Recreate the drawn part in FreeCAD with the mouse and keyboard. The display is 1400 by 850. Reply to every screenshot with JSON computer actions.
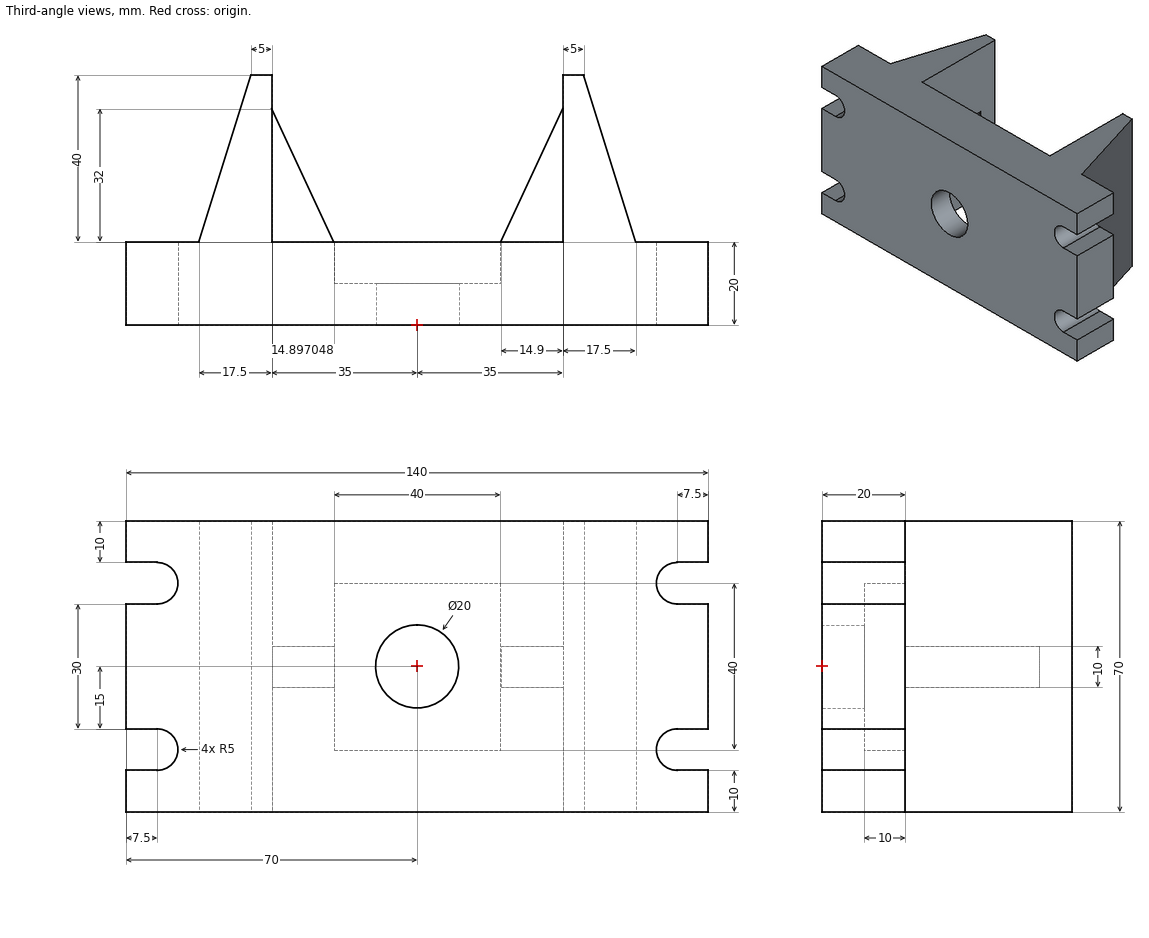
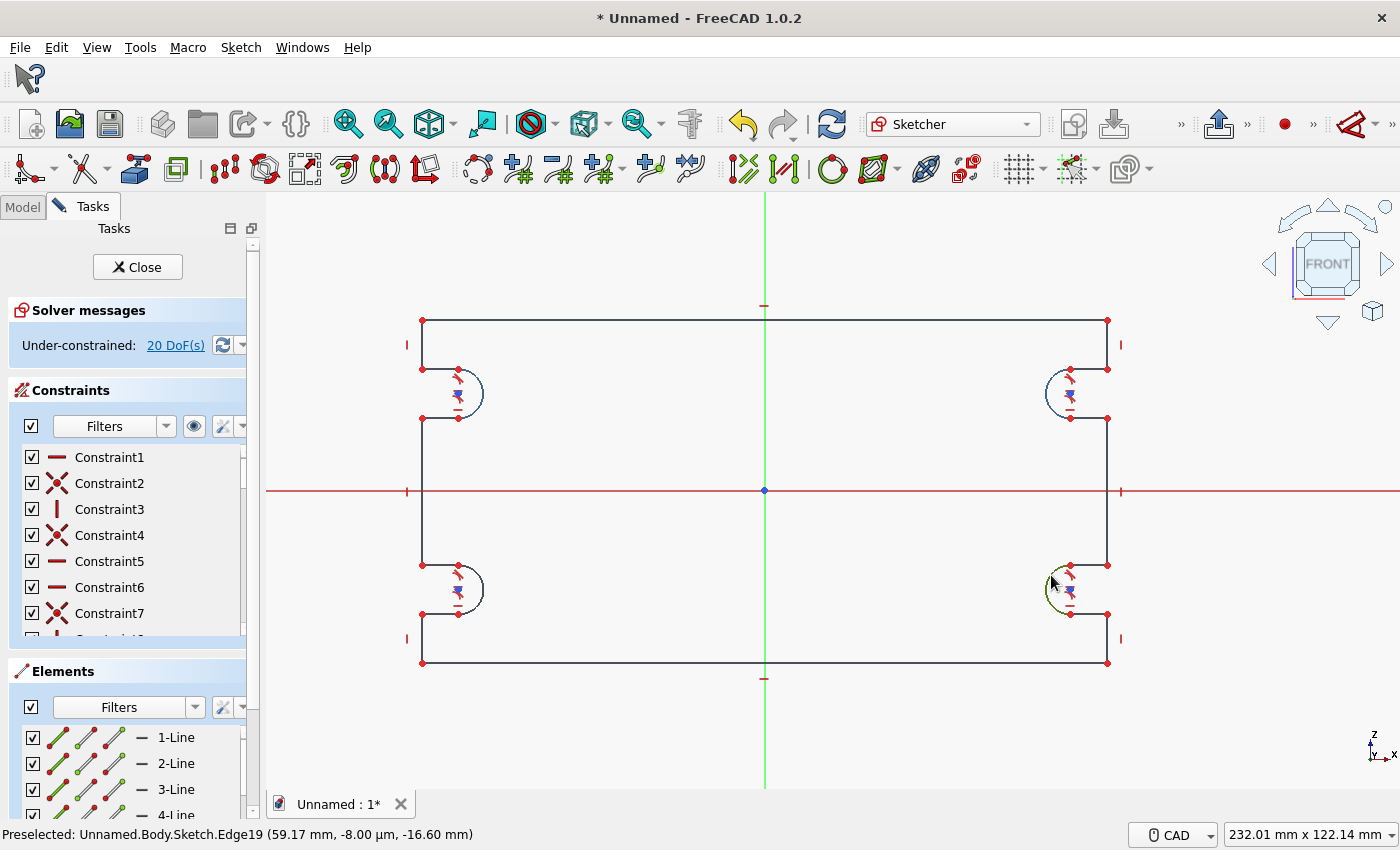
{"action": "left_click", "coordinate": [479, 604]}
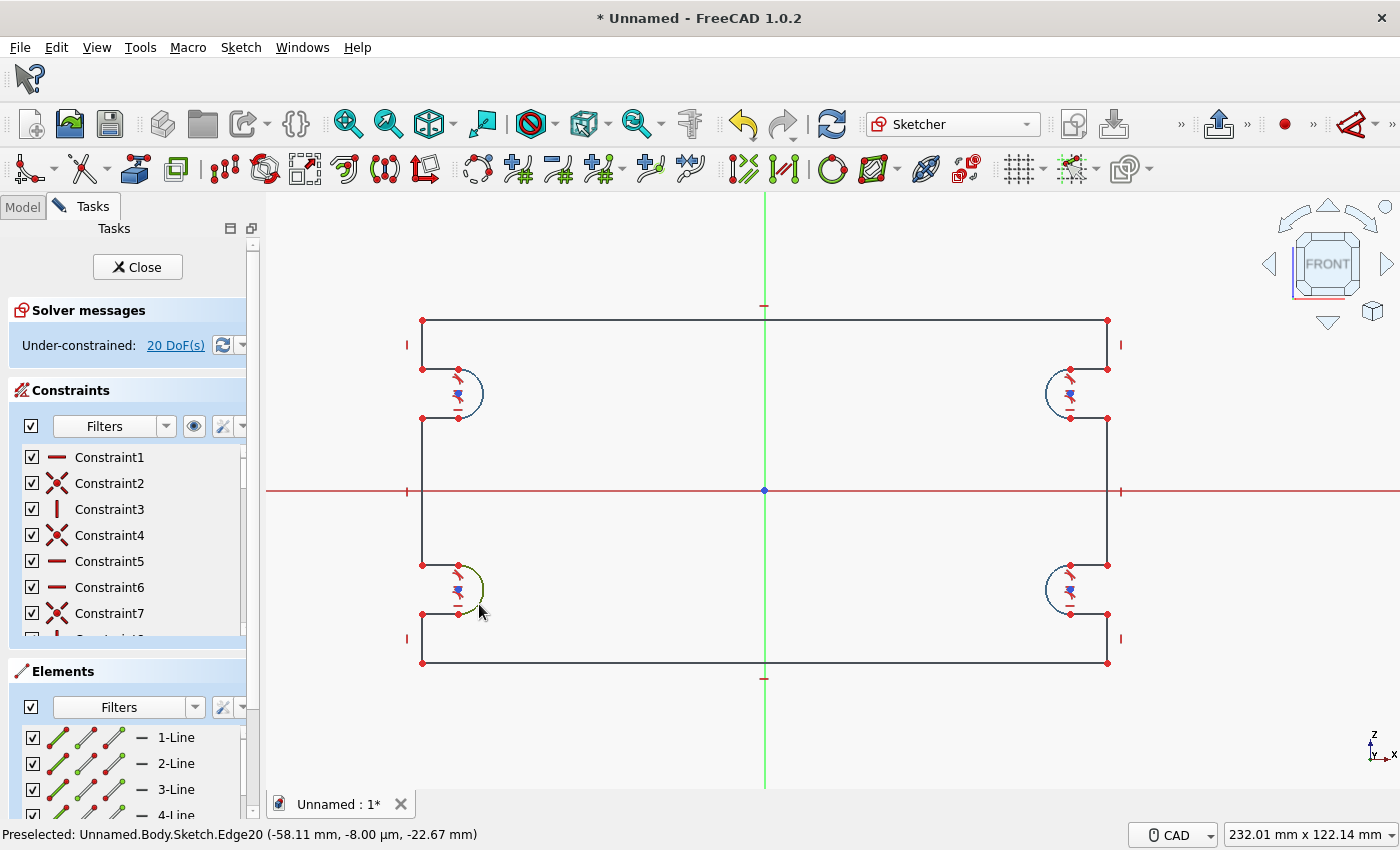
{"action": "key", "text": "e"}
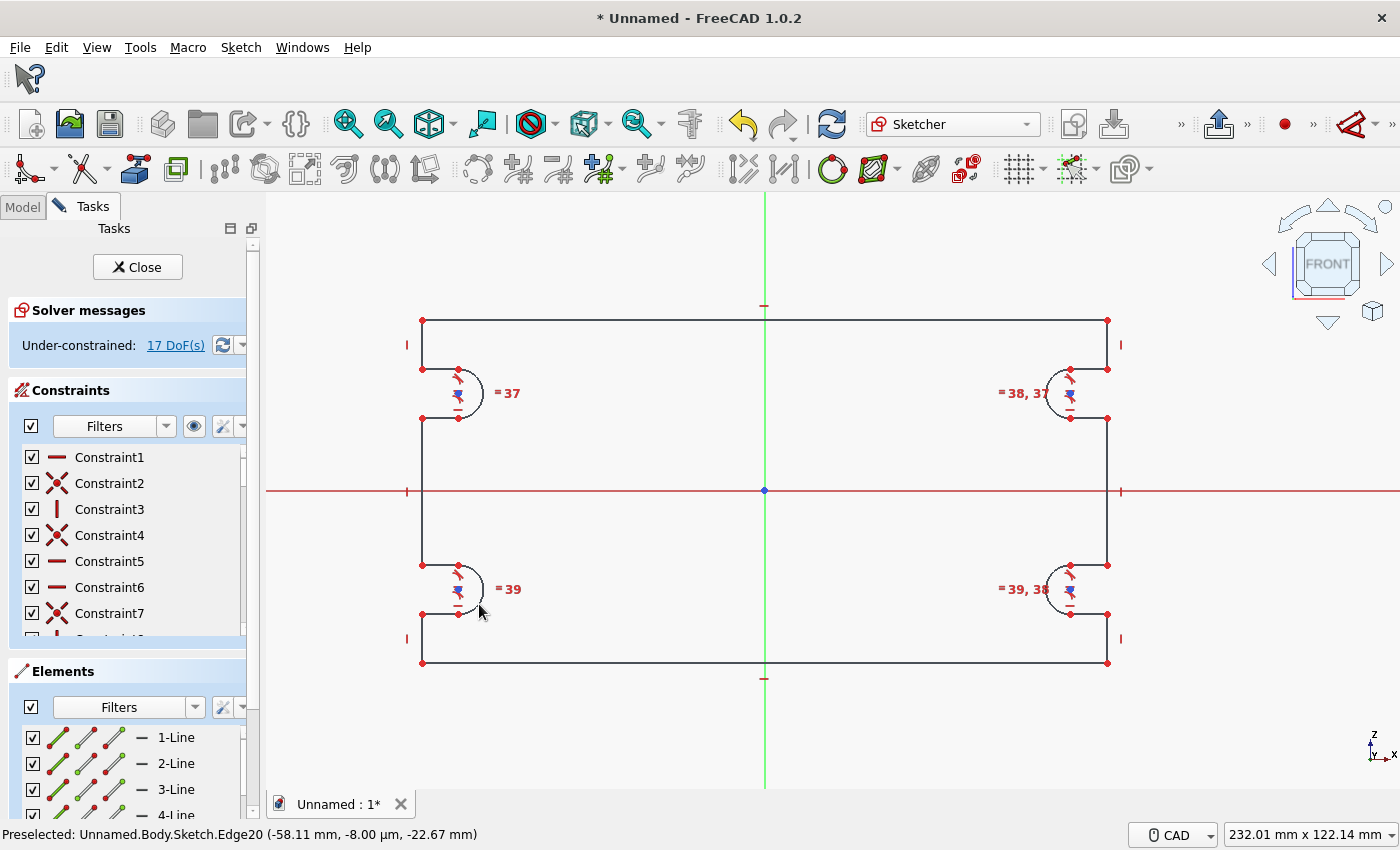
{"action": "scroll", "coordinate": [478, 408], "scroll_direction": "up", "scroll_amount": 3}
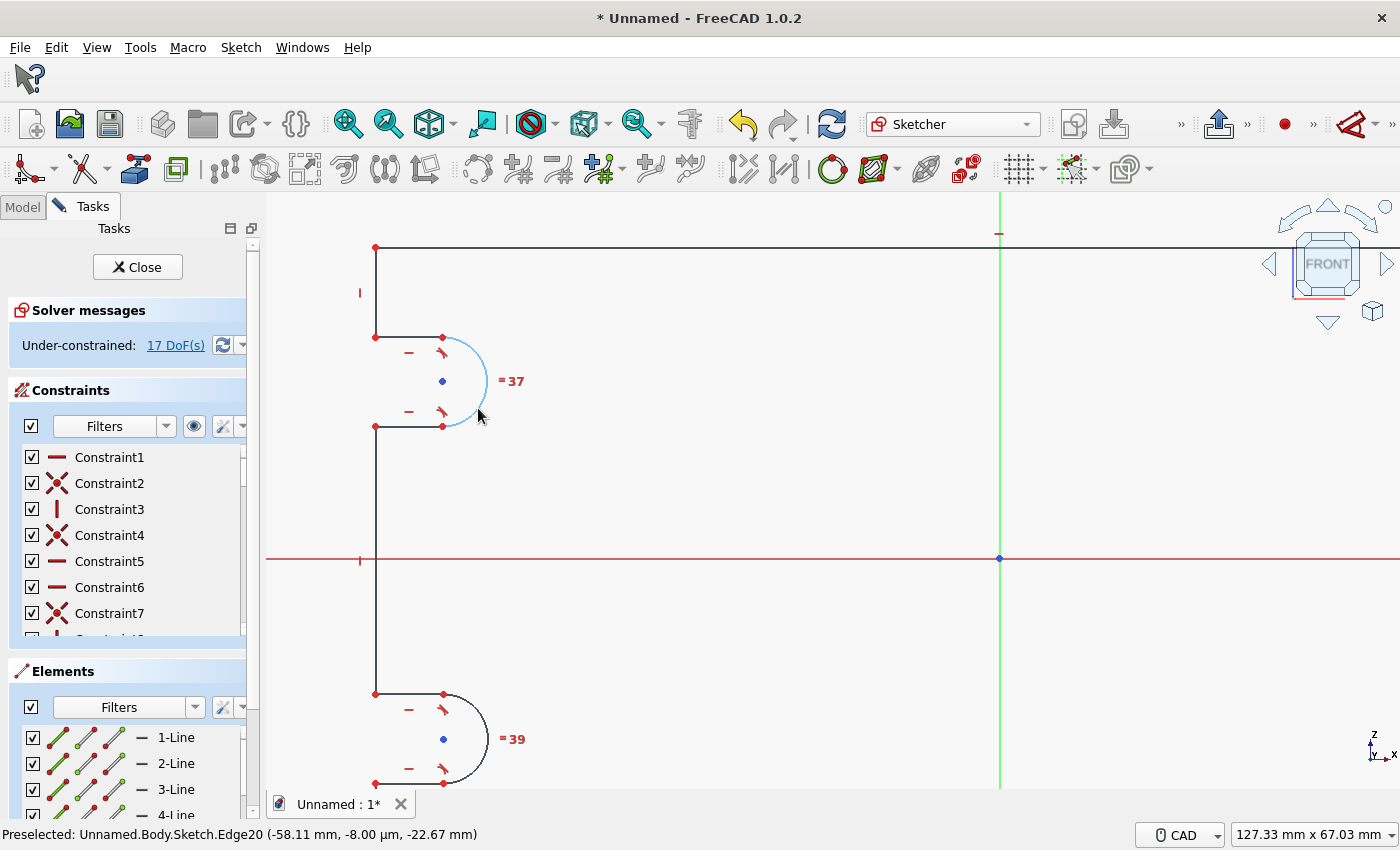
{"action": "left_click", "coordinate": [478, 408]}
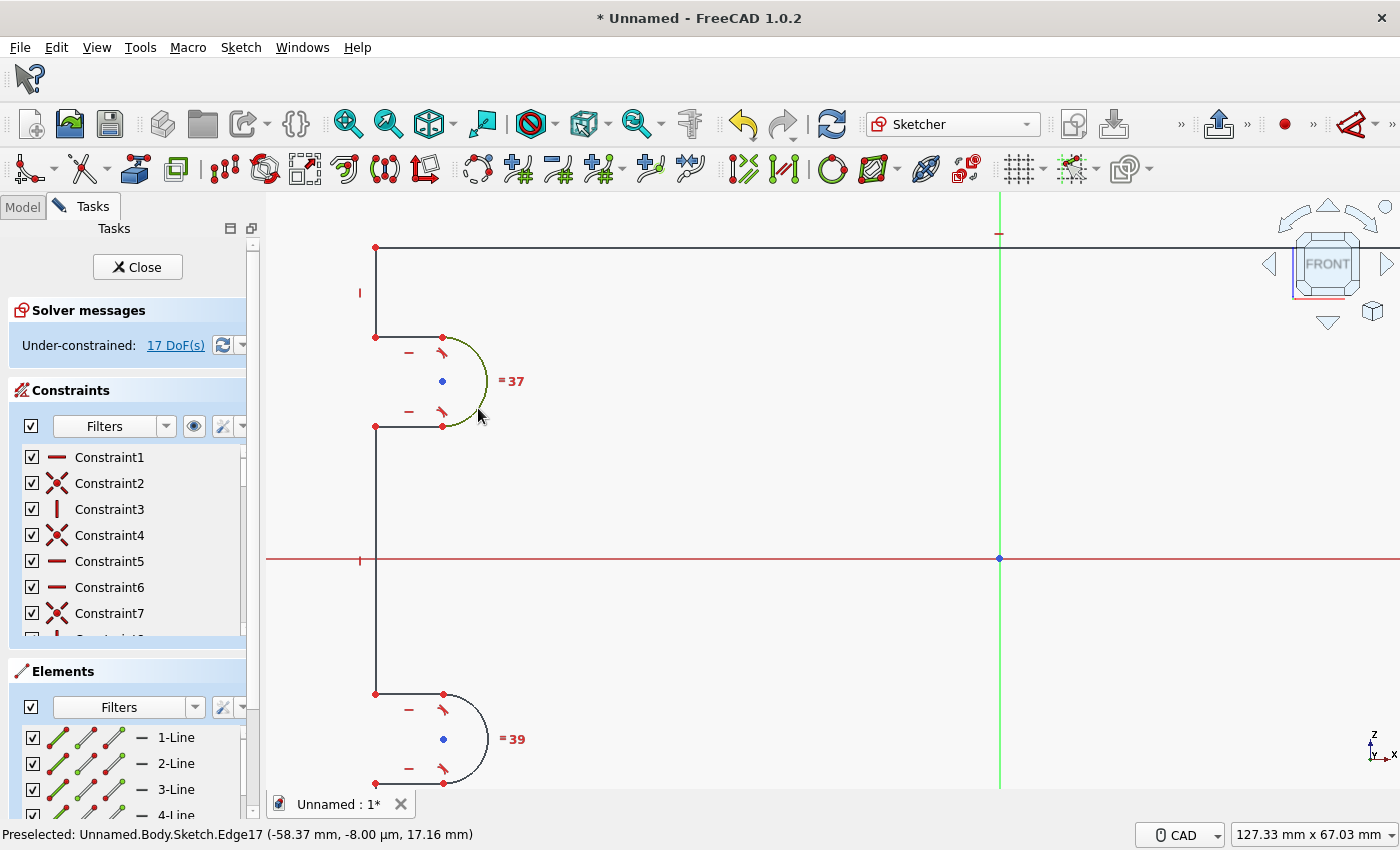
{"action": "left_click", "coordinate": [1378, 124]}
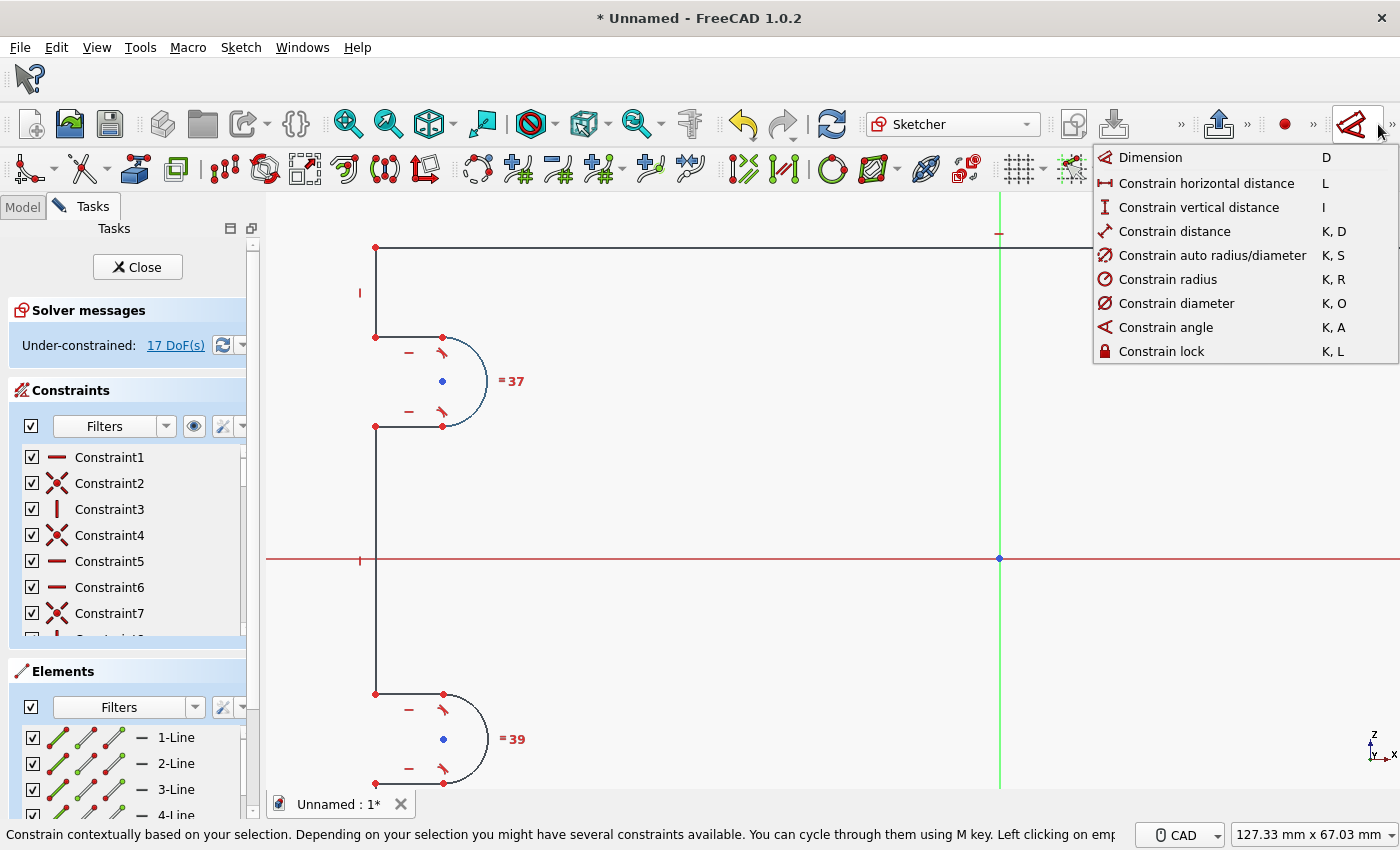
{"action": "left_click", "coordinate": [1246, 279]}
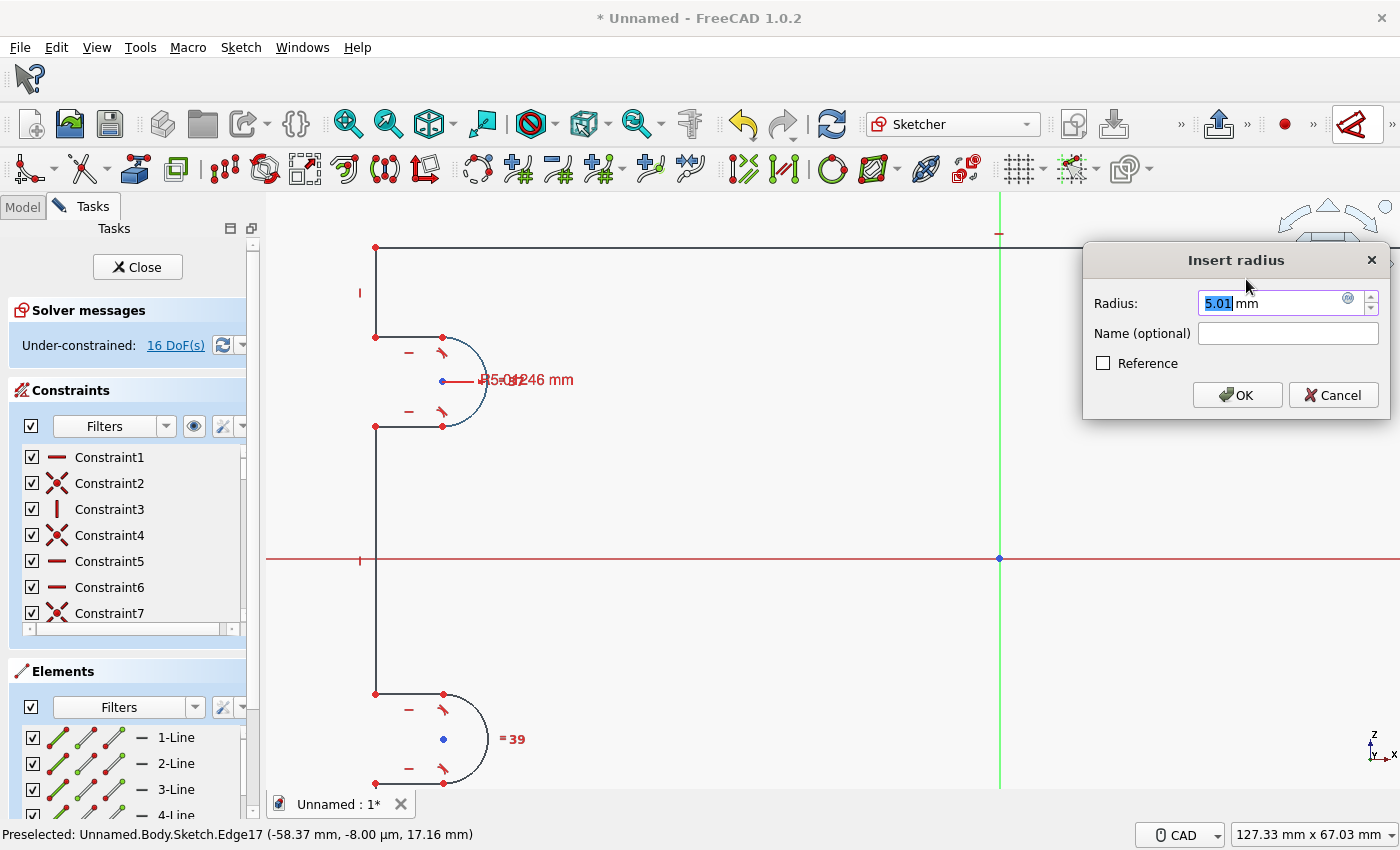
{"action": "type", "text": "5"}
{"action": "key", "text": "Return"}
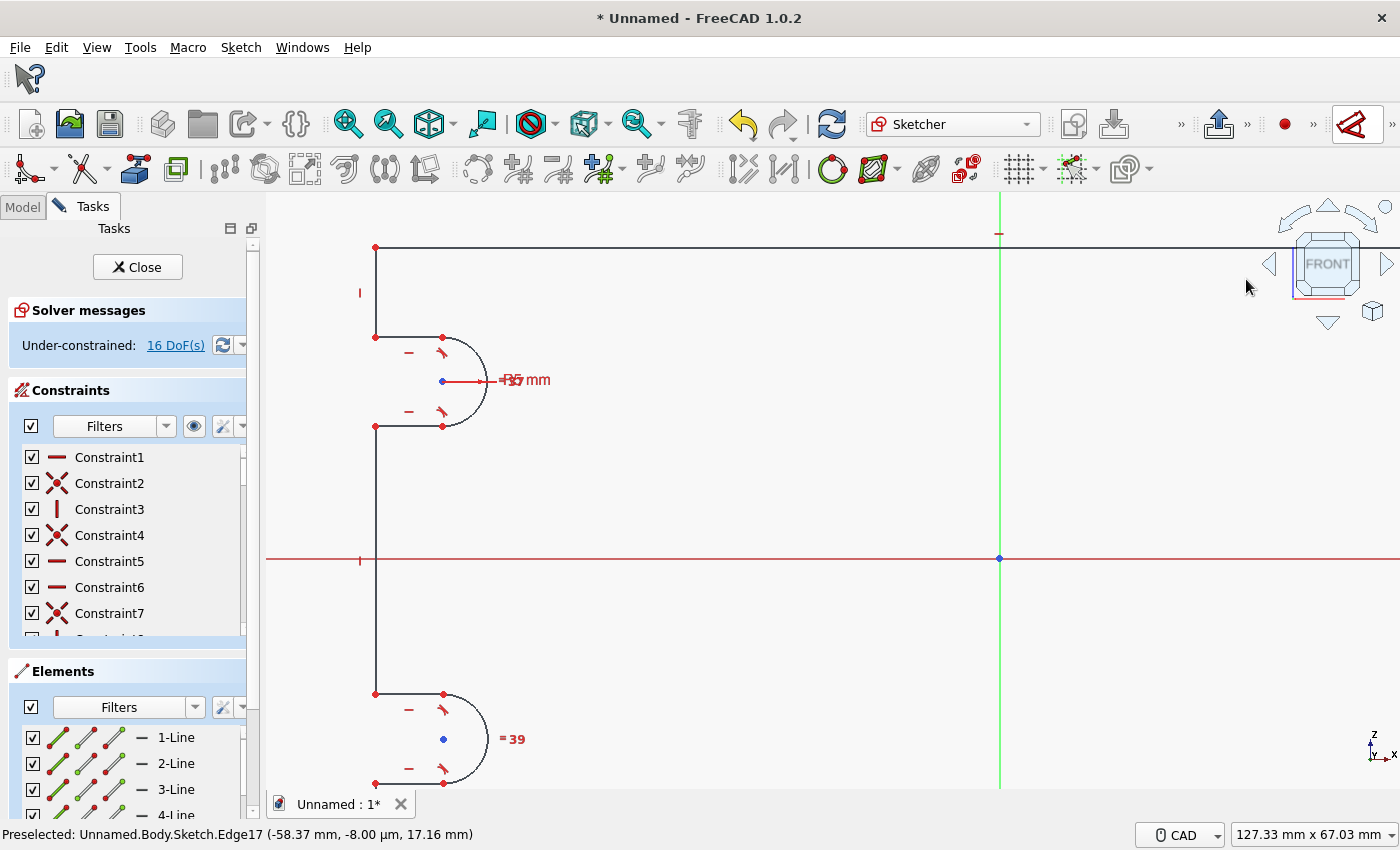
{"action": "left_click", "coordinate": [376, 614]}